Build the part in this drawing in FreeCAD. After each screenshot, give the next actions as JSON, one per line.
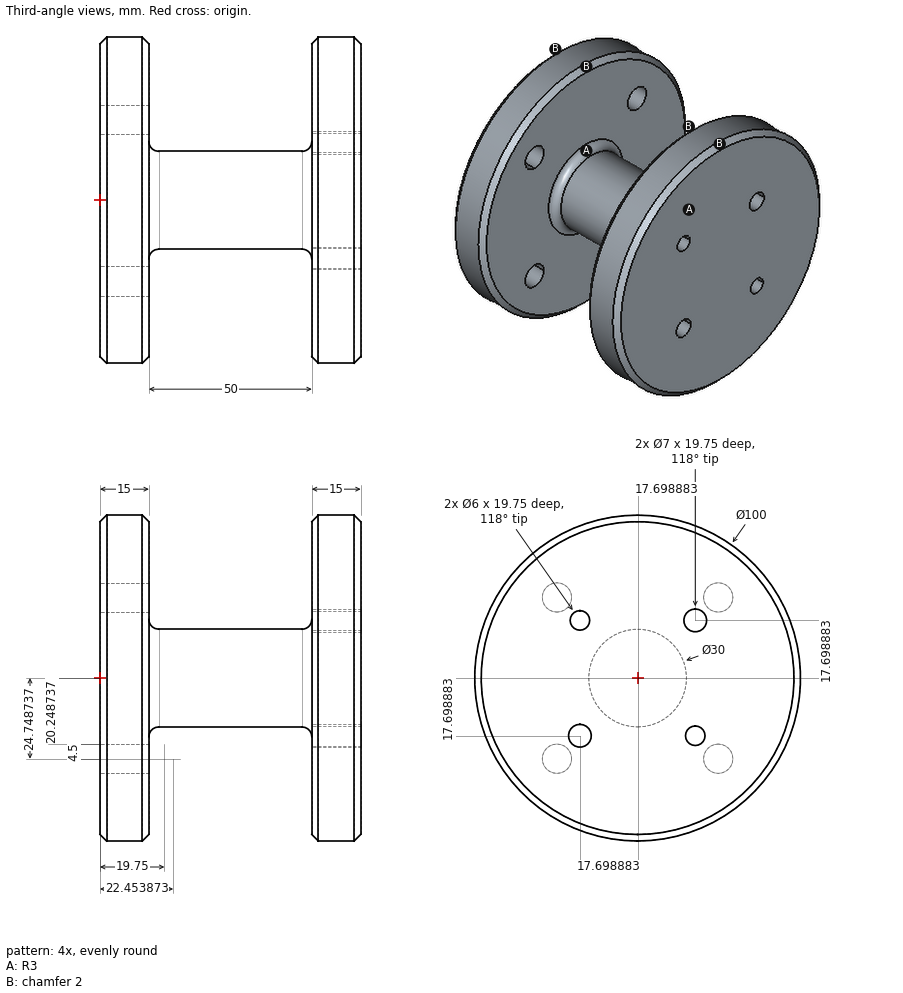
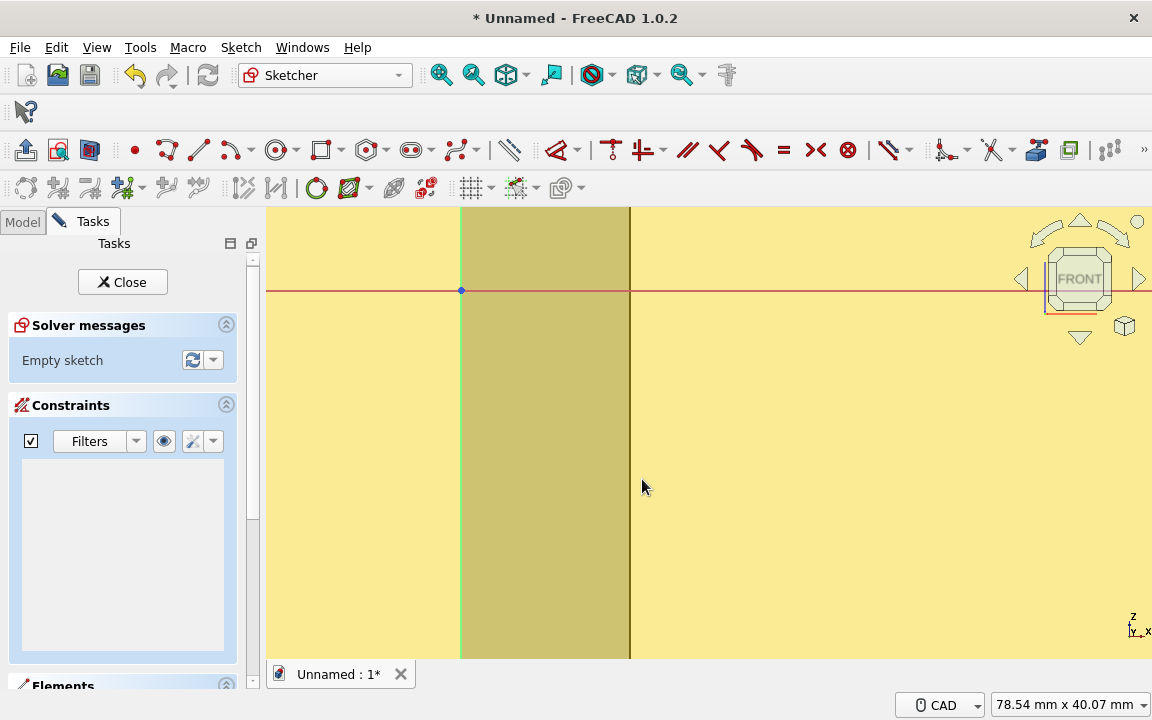
{"action": "left_click", "coordinate": [168, 150]}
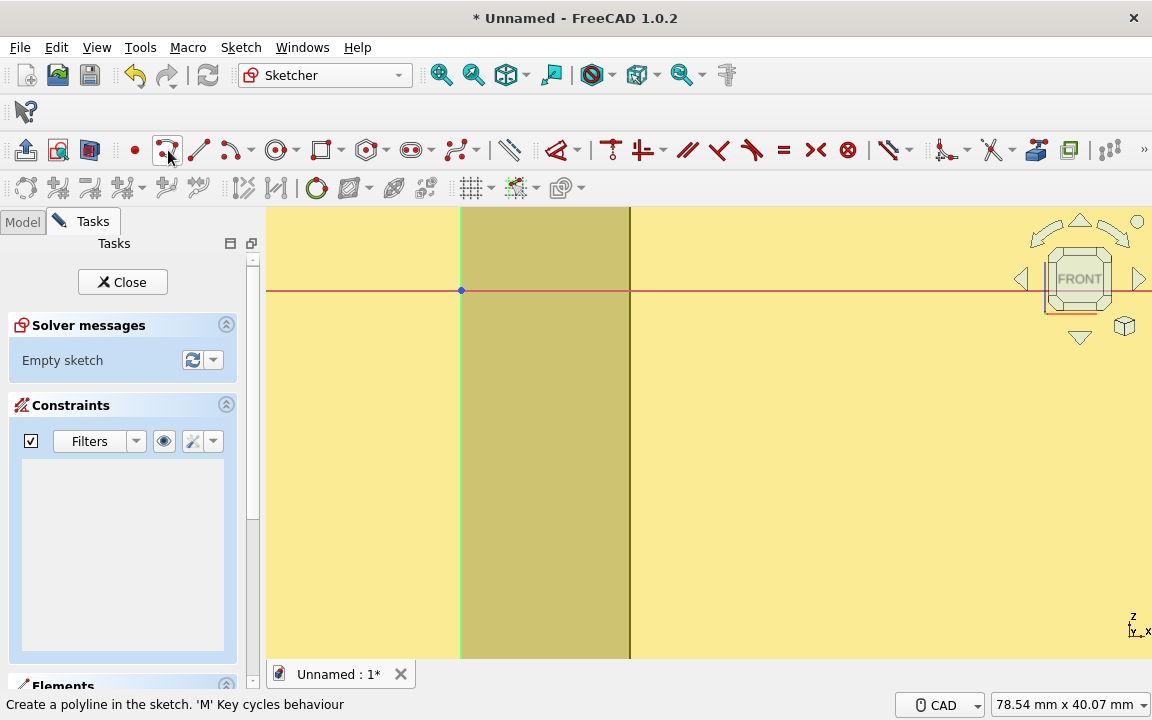
{"action": "left_click", "coordinate": [461, 519]}
{"action": "left_click", "coordinate": [684, 519]}
{"action": "left_click", "coordinate": [714, 570]}
{"action": "left_click", "coordinate": [470, 570]}
{"action": "left_click", "coordinate": [461, 520]}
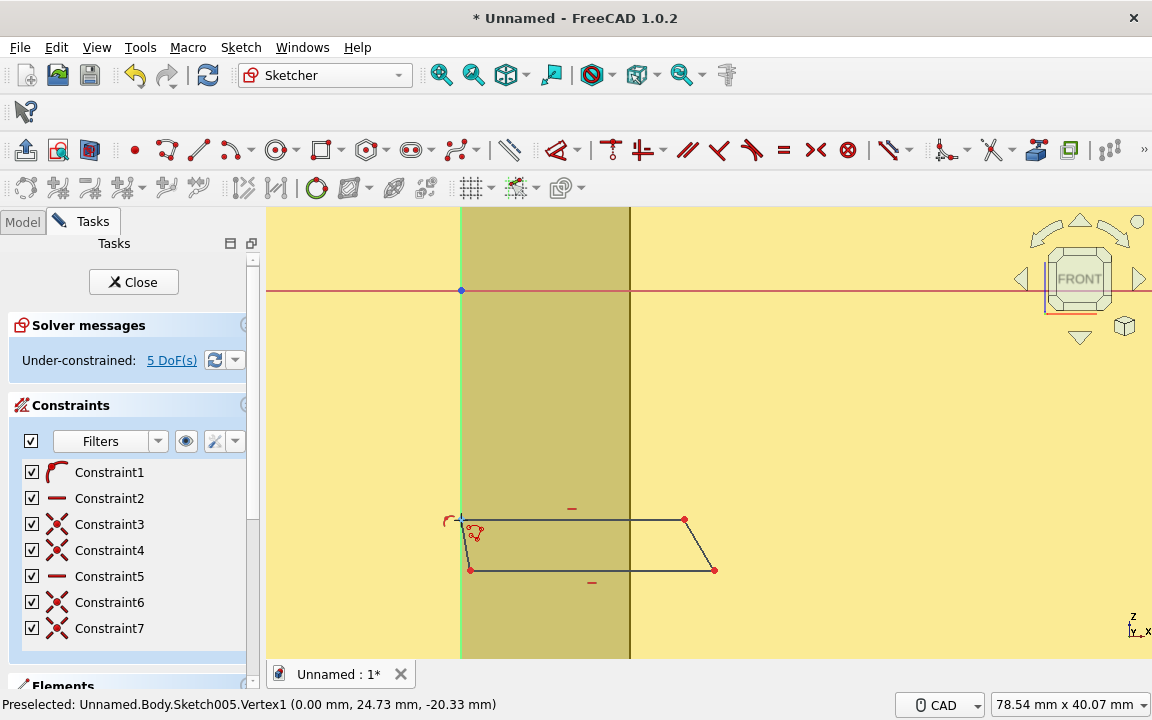
{"action": "left_click", "coordinate": [200, 150]}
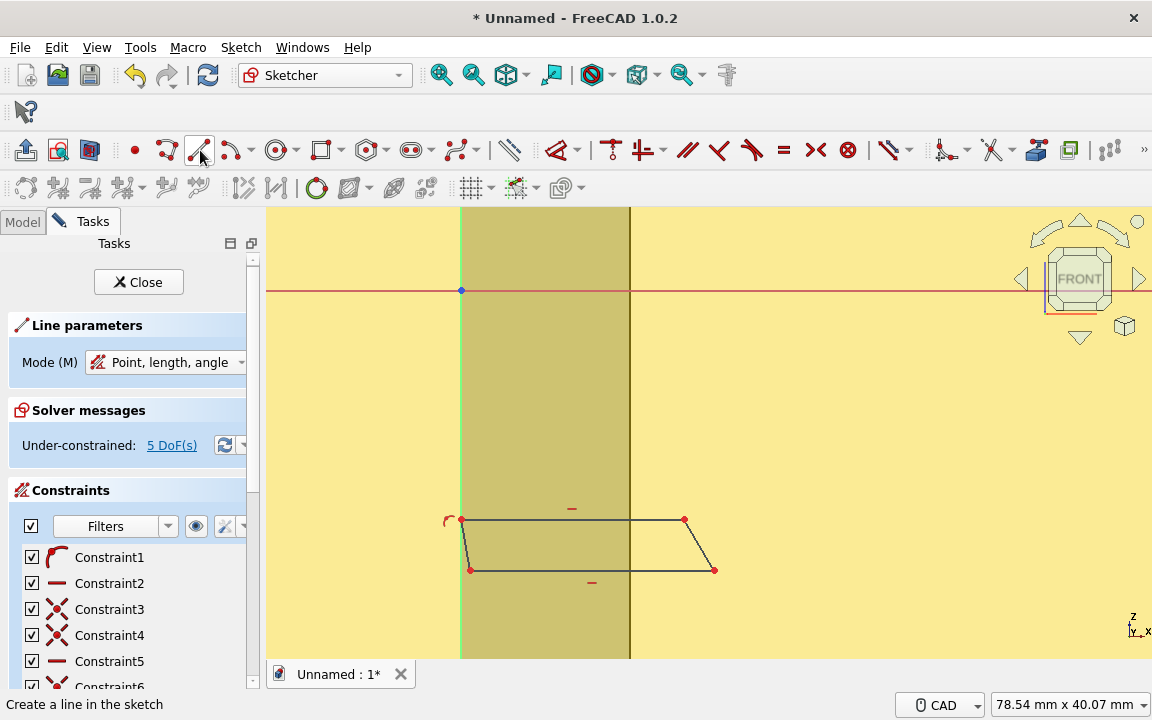
{"action": "left_click", "coordinate": [740, 570]}
{"action": "left_click", "coordinate": [816, 570]}
{"action": "key", "text": "Escape"}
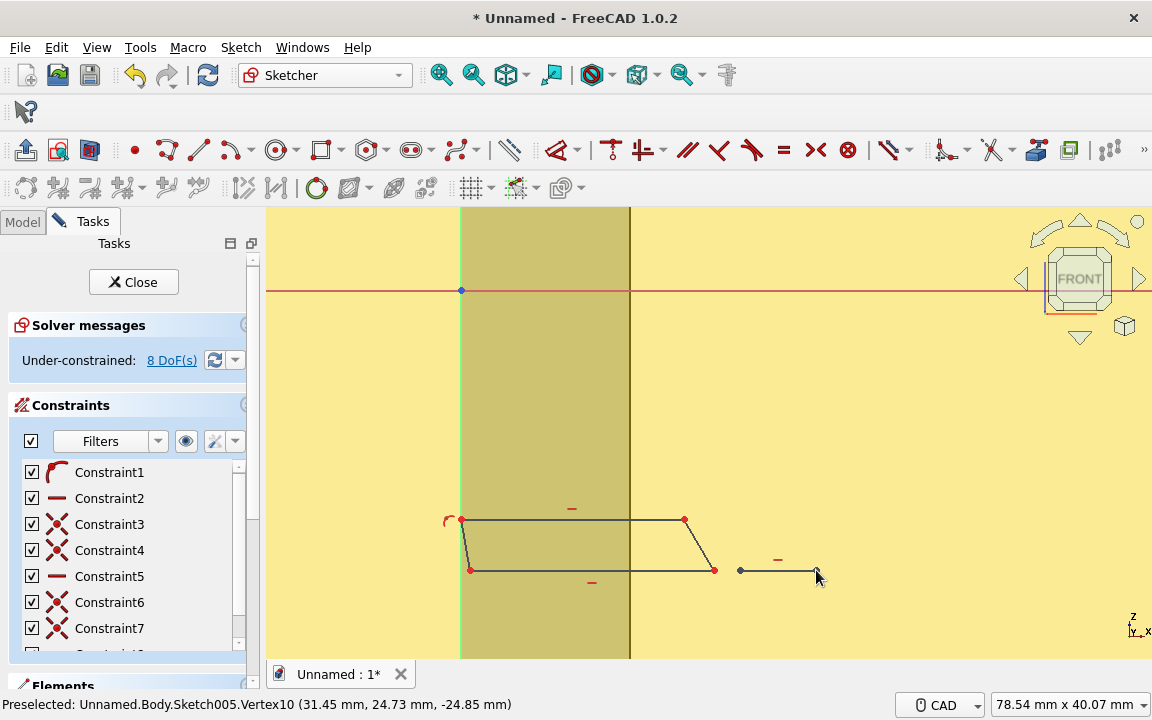
{"action": "left_click", "coordinate": [763, 571]}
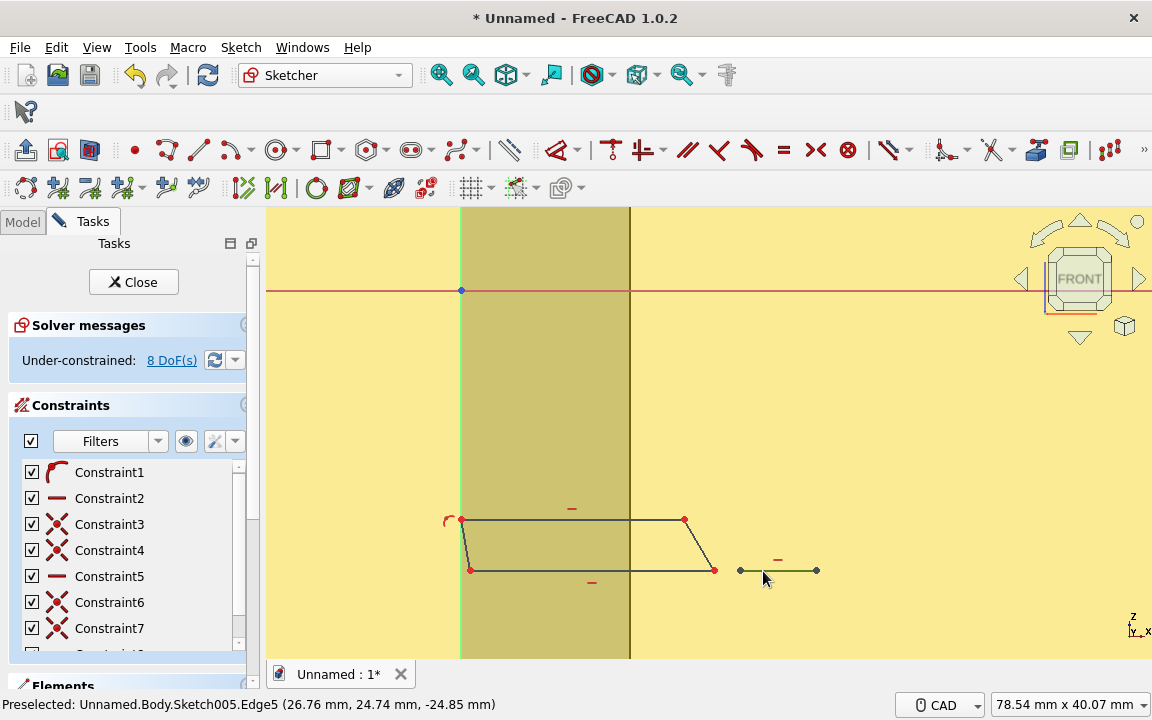
{"action": "left_click", "coordinate": [510, 150]}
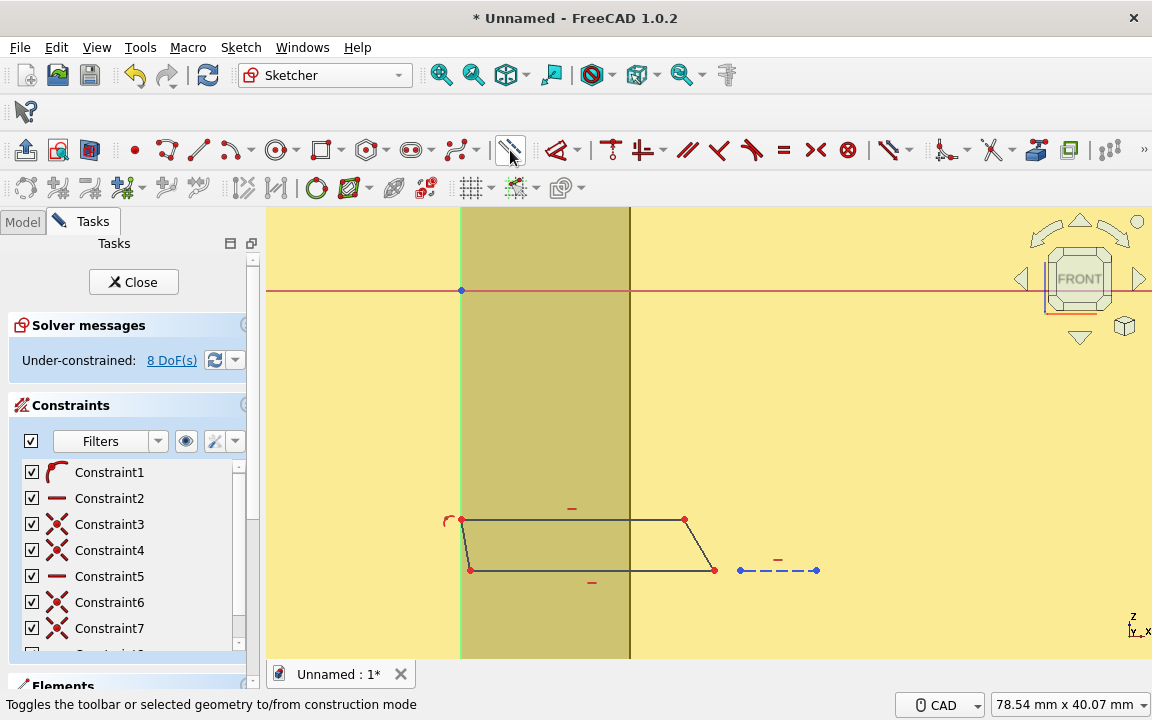
{"action": "left_click", "coordinate": [464, 535]}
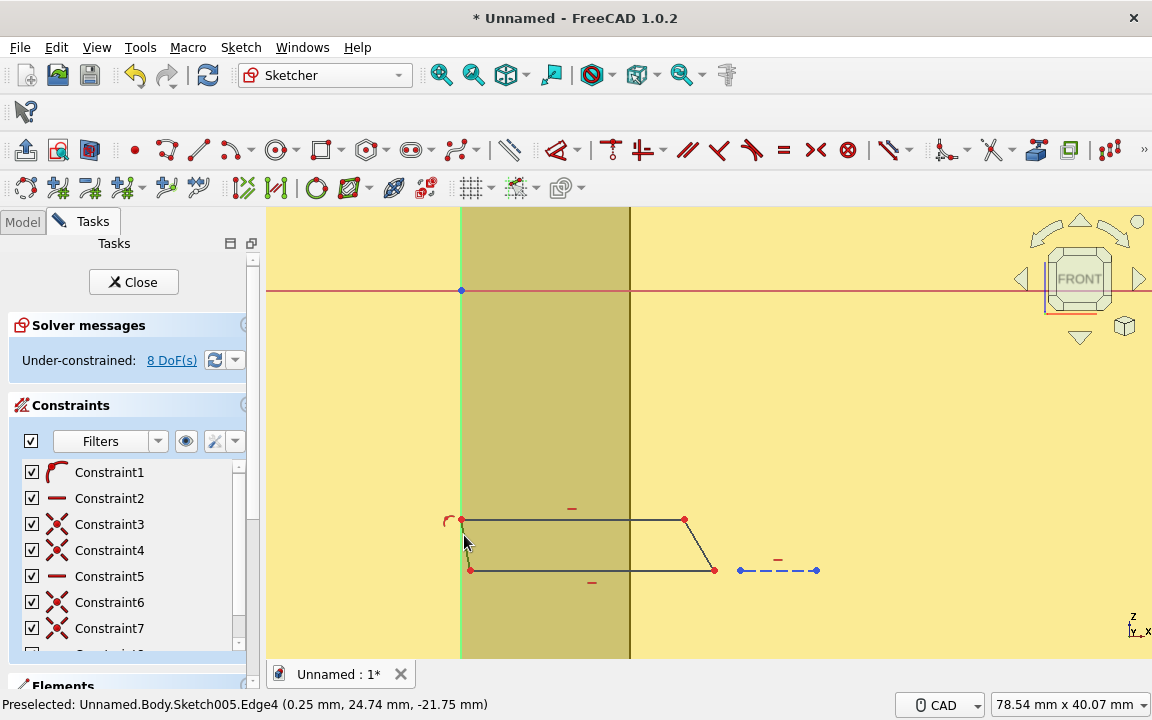
{"action": "left_click", "coordinate": [666, 150]}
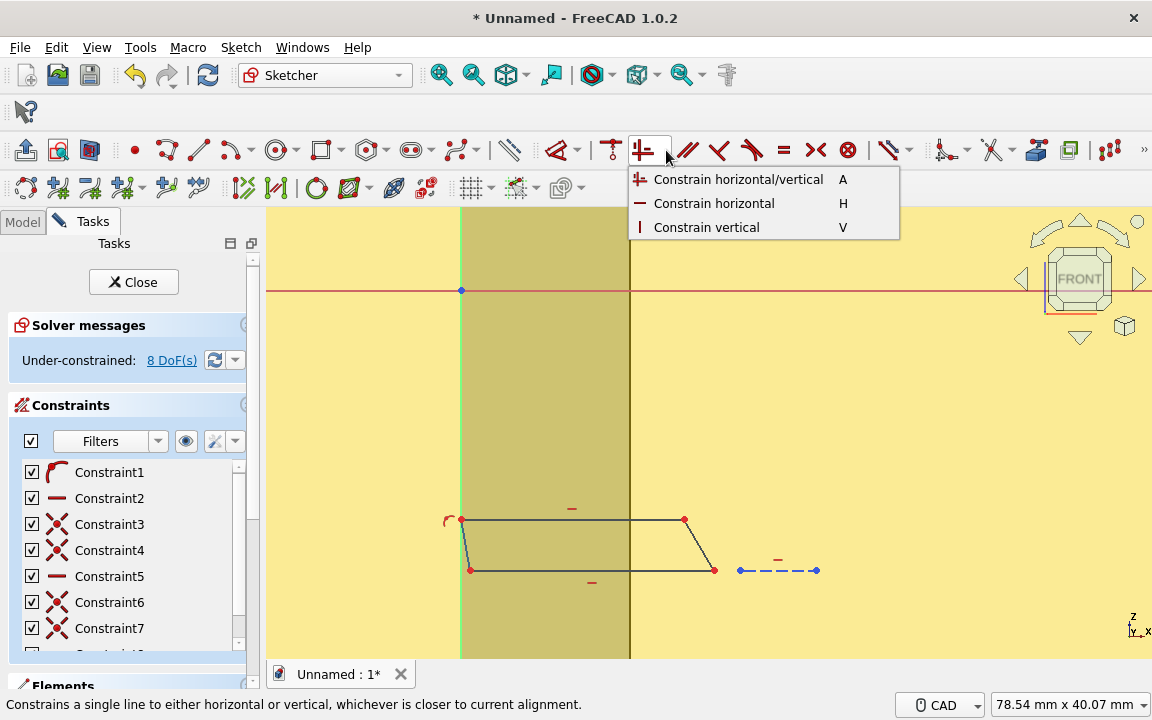
{"action": "left_click", "coordinate": [764, 227]}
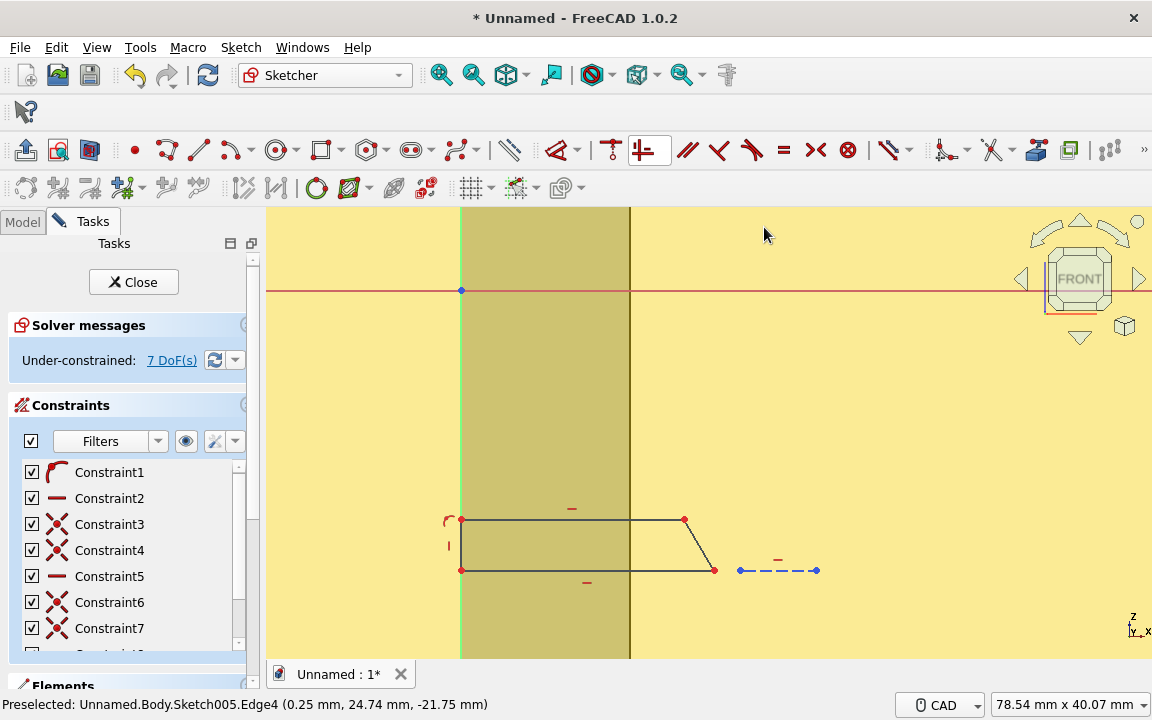
{"action": "left_click", "coordinate": [556, 150]}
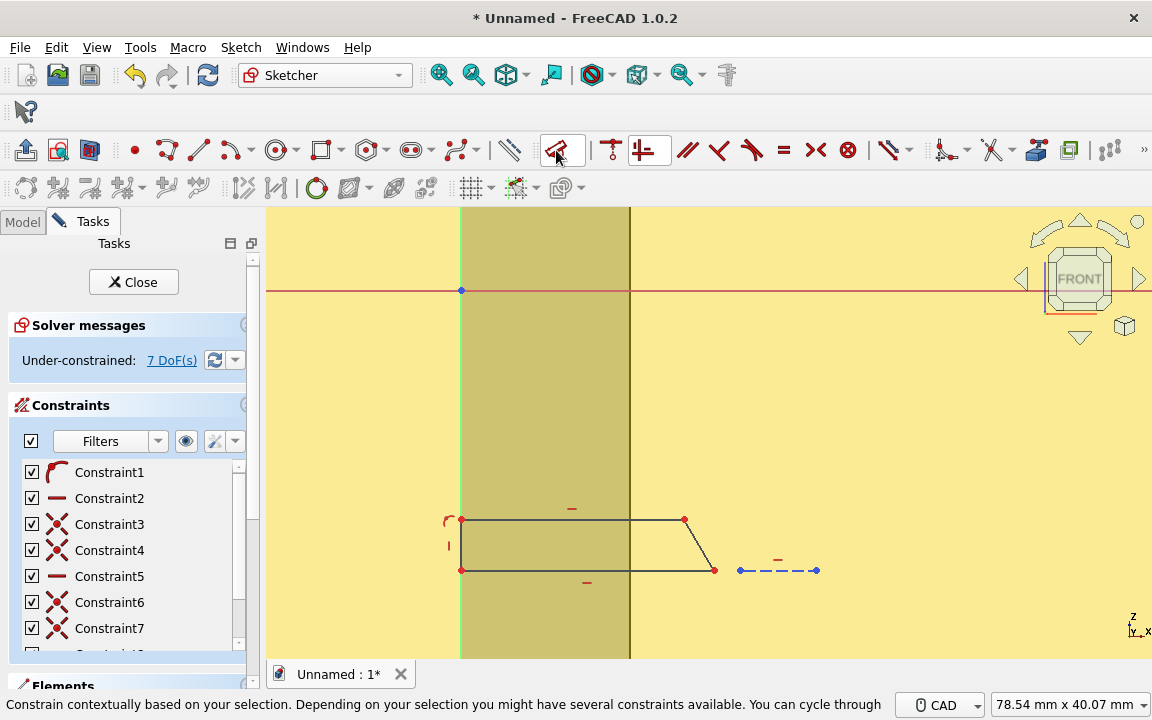
{"action": "left_click", "coordinate": [461, 556]}
{"action": "left_click", "coordinate": [427, 545]}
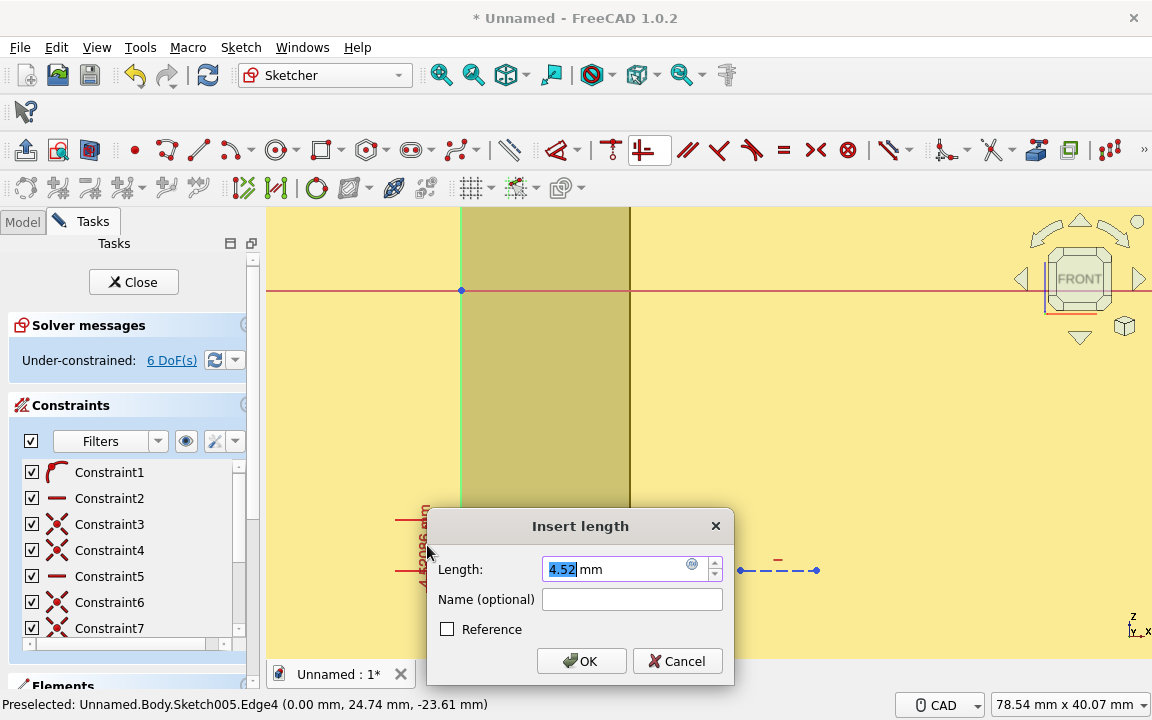
{"action": "type", "text": "4.5"}
{"action": "key", "text": "Return"}